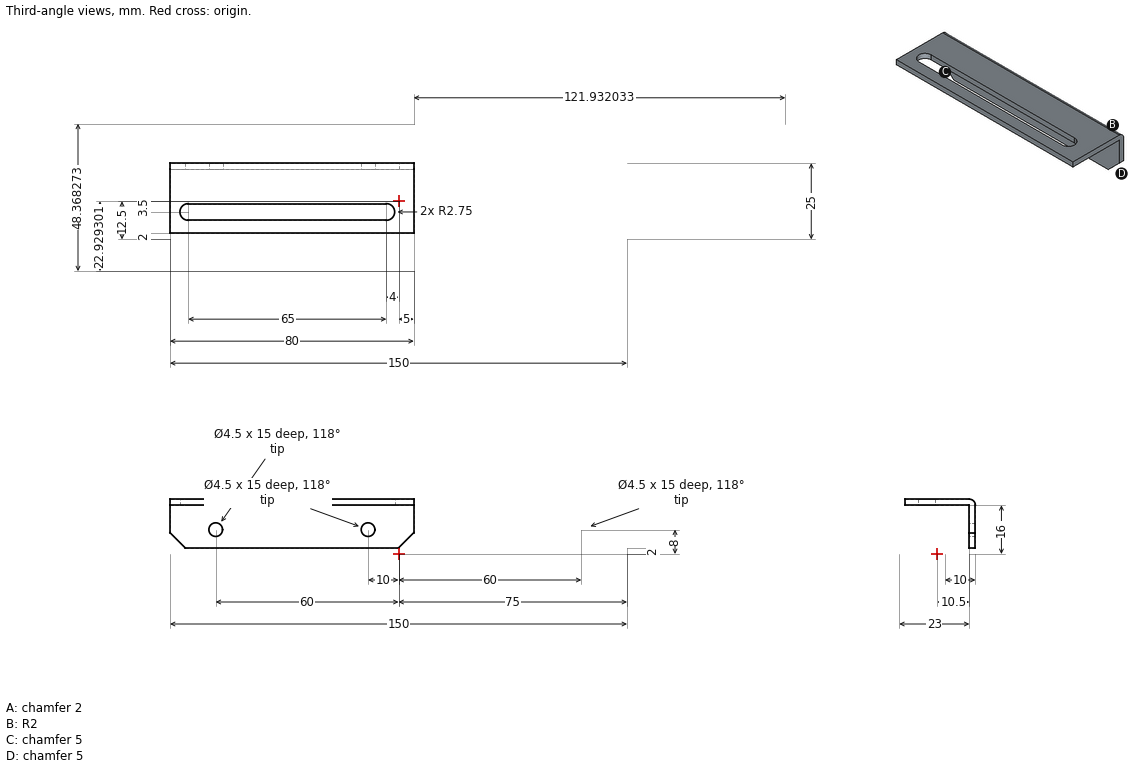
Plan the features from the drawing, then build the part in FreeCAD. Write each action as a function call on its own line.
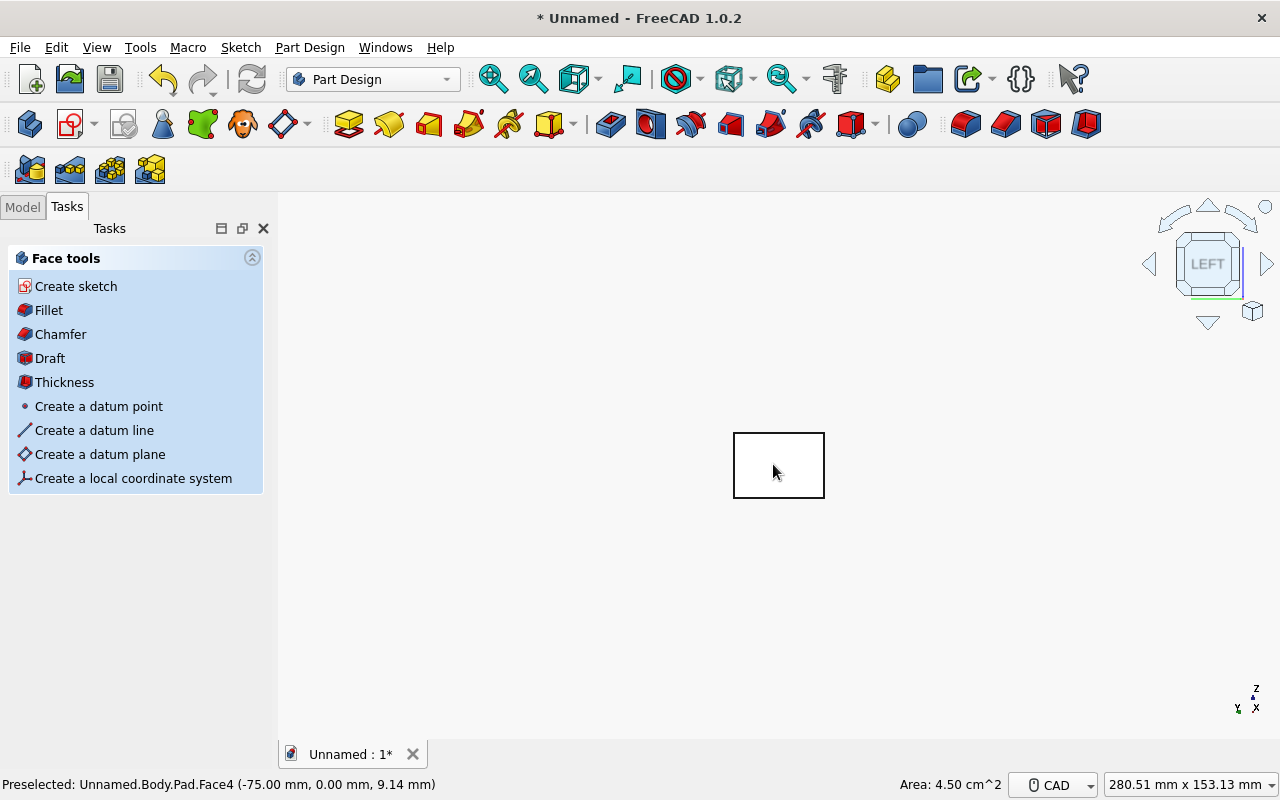
click(70, 124)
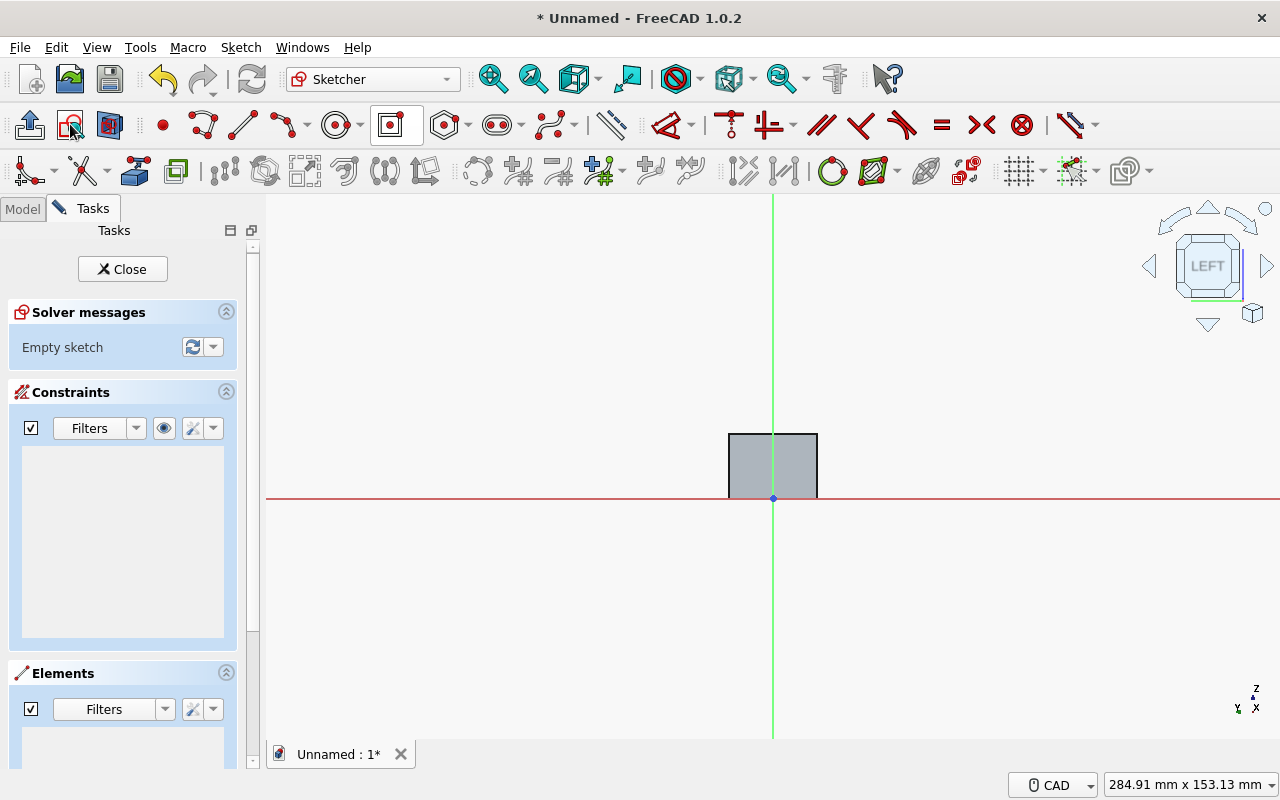
scroll(791, 471, up, 9)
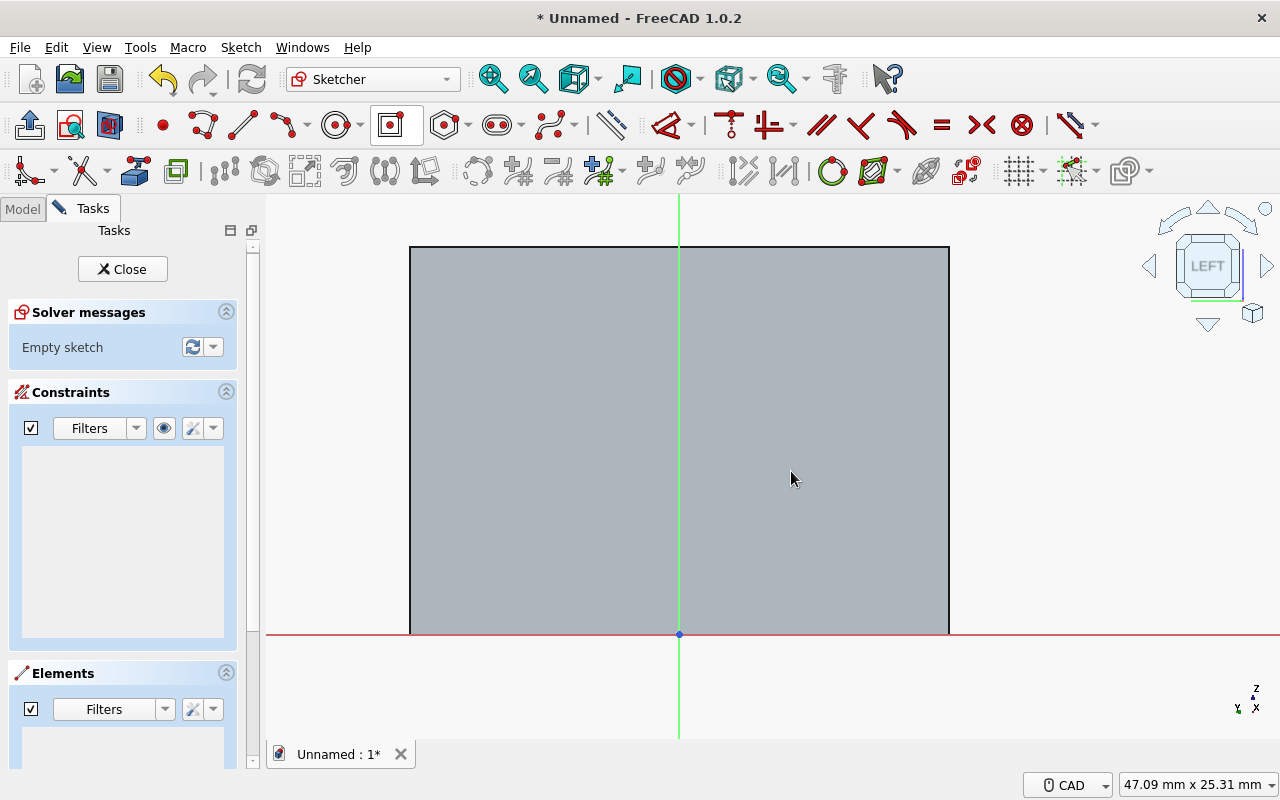
key(g)
key(r)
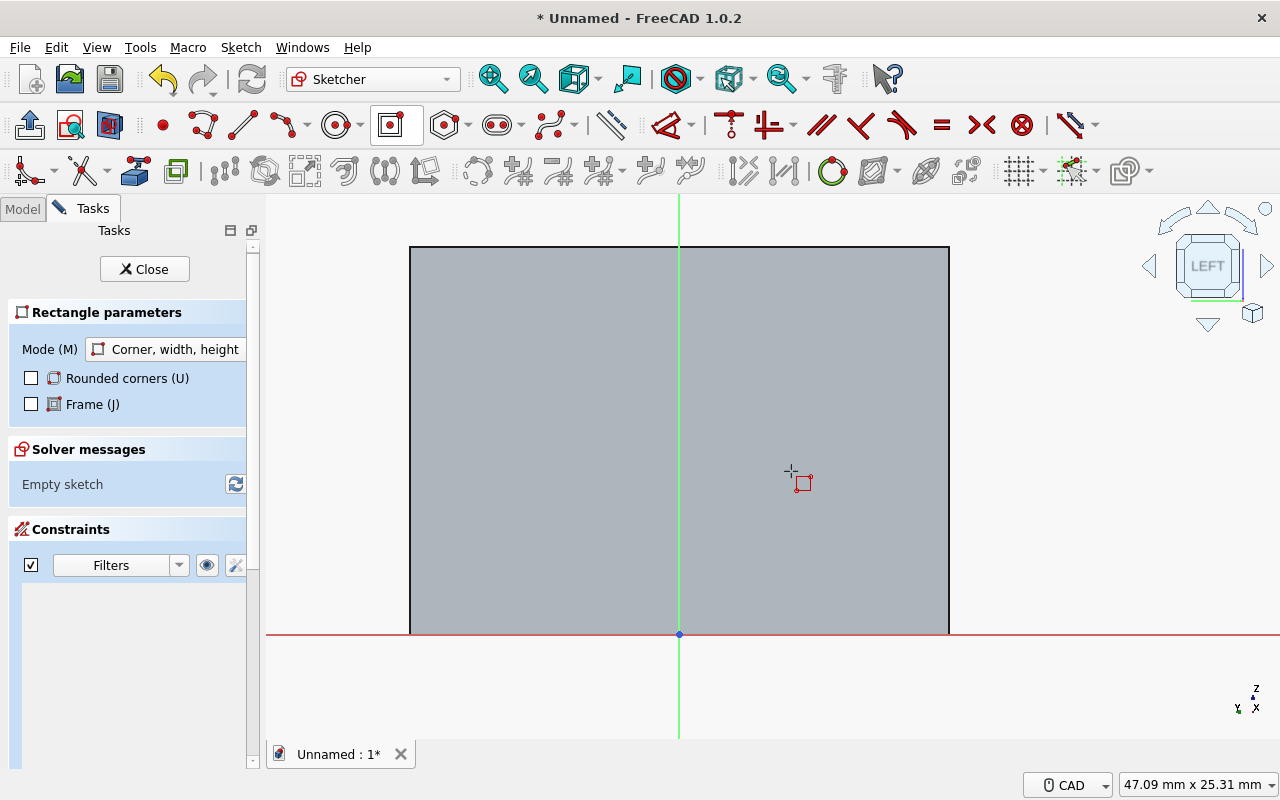
click(453, 290)
click(949, 635)
key(Escape)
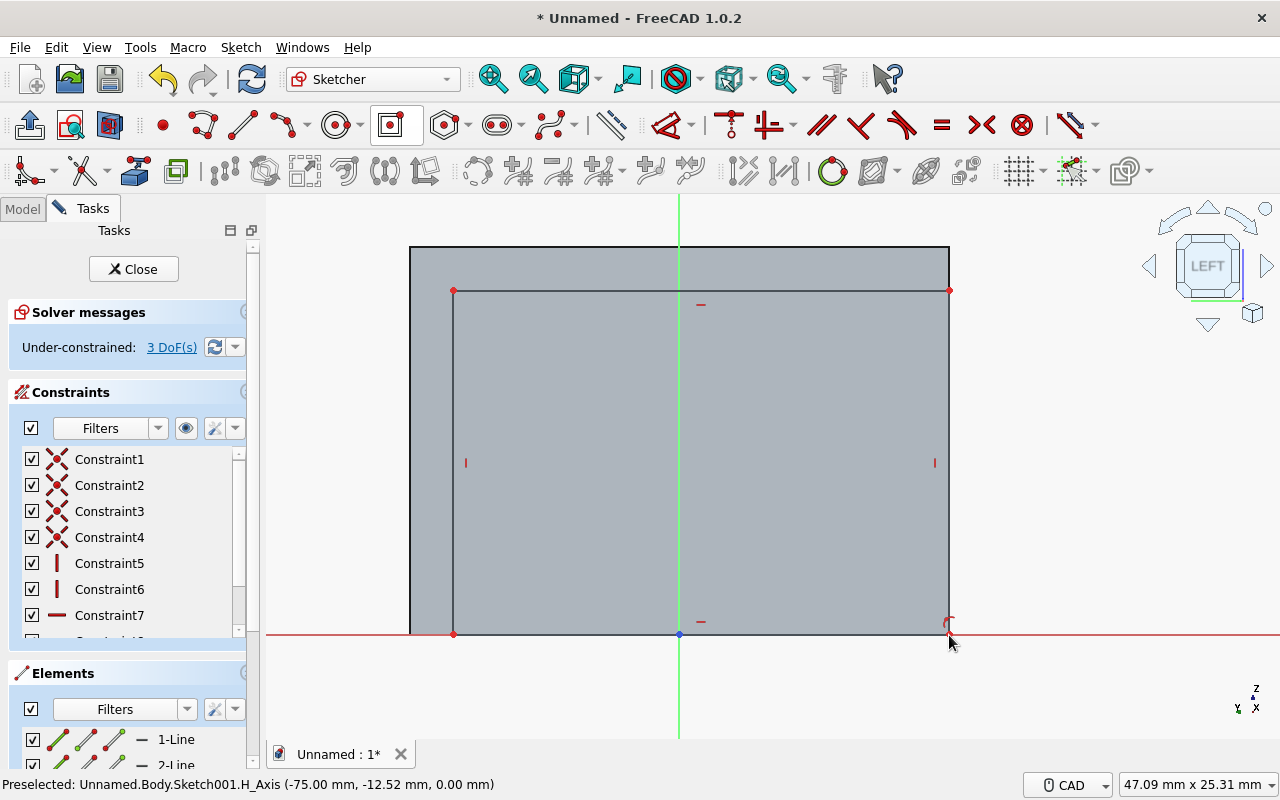
click(666, 126)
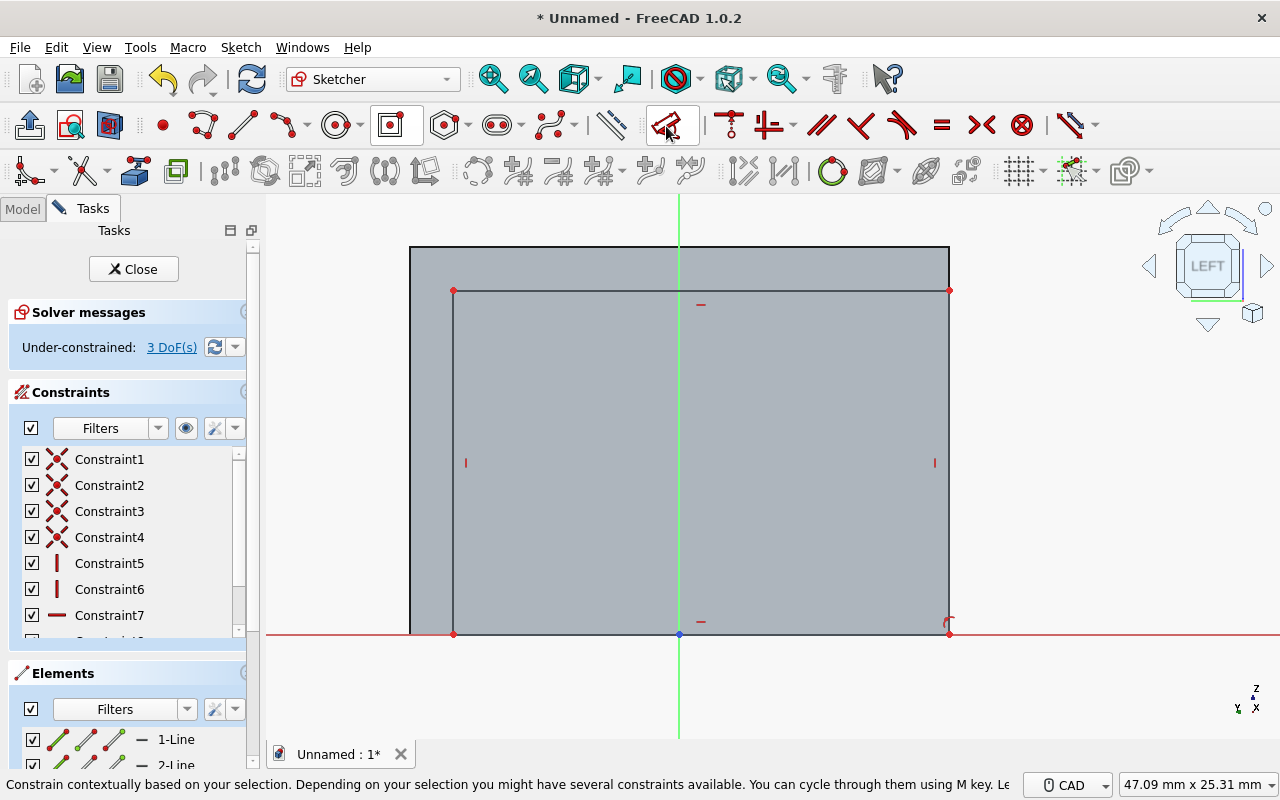
click(453, 394)
click(419, 463)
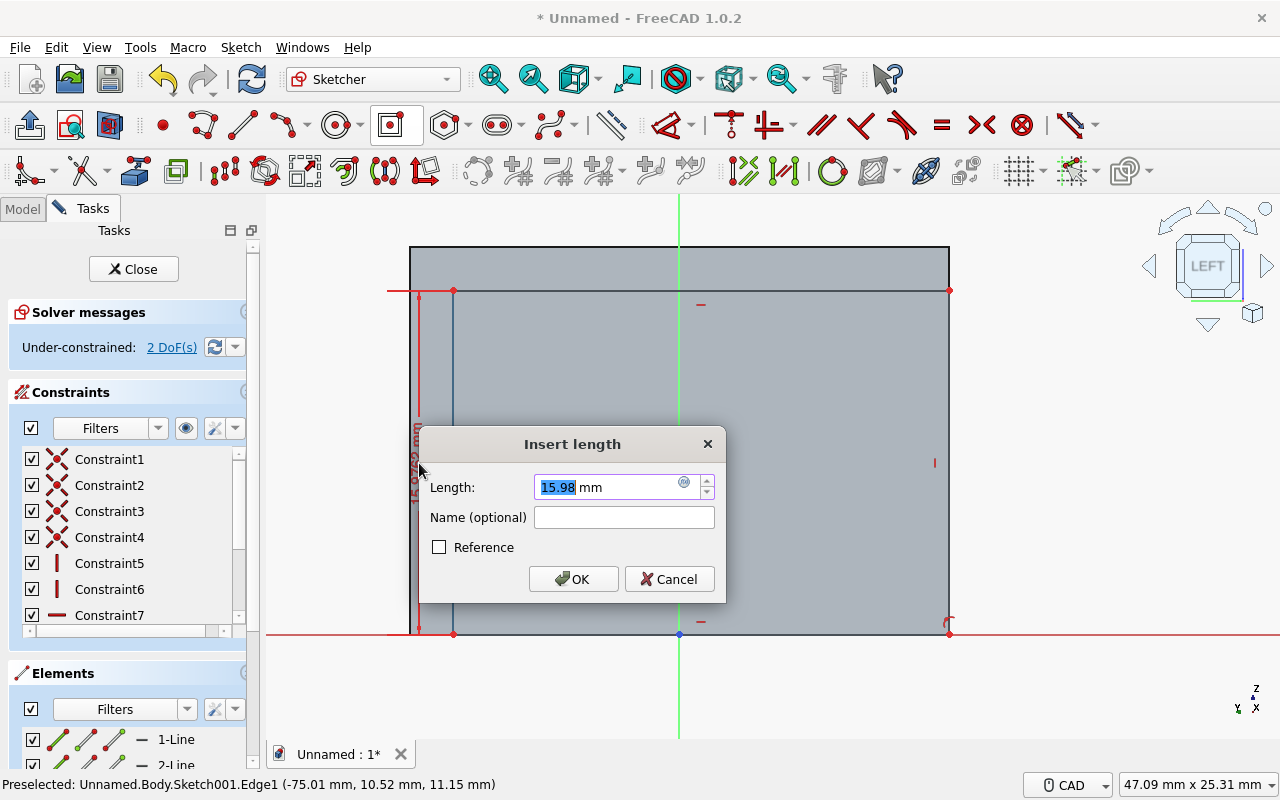
text(16)
key(Return)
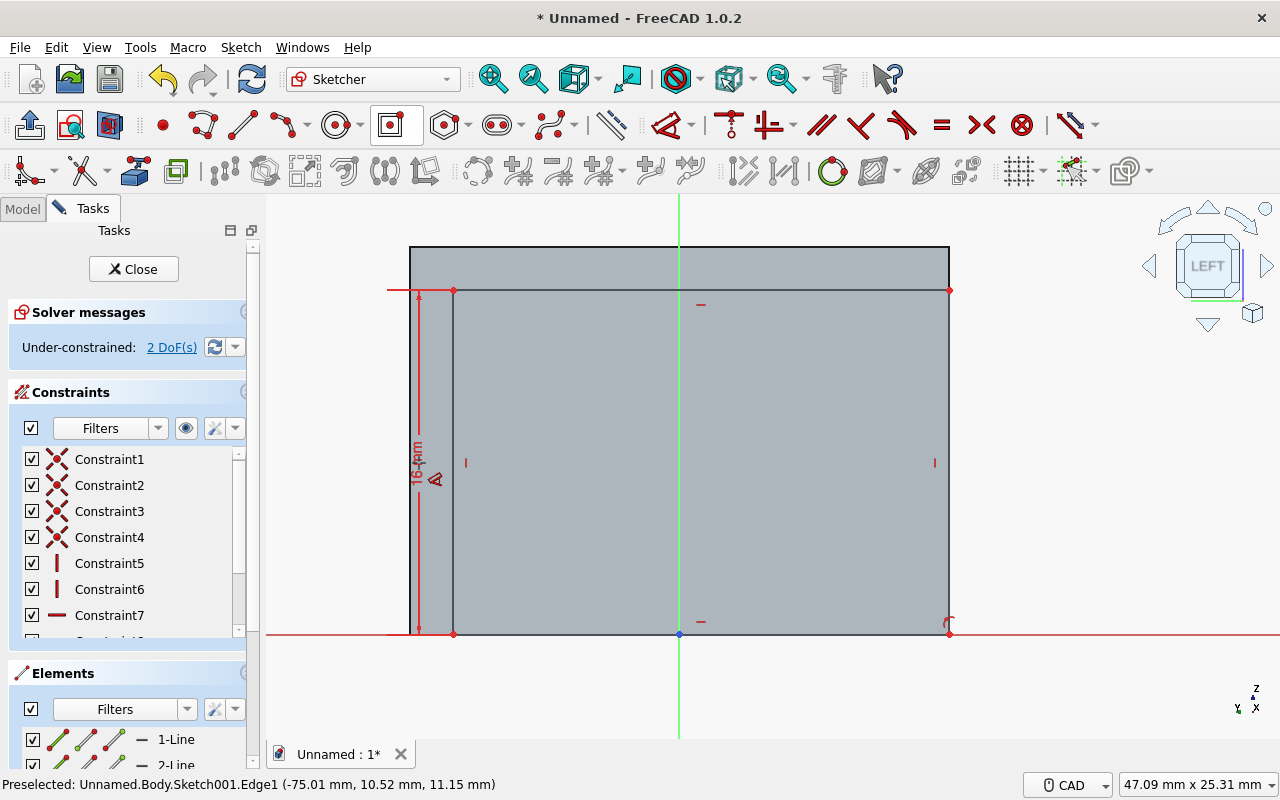
click(602, 635)
click(701, 669)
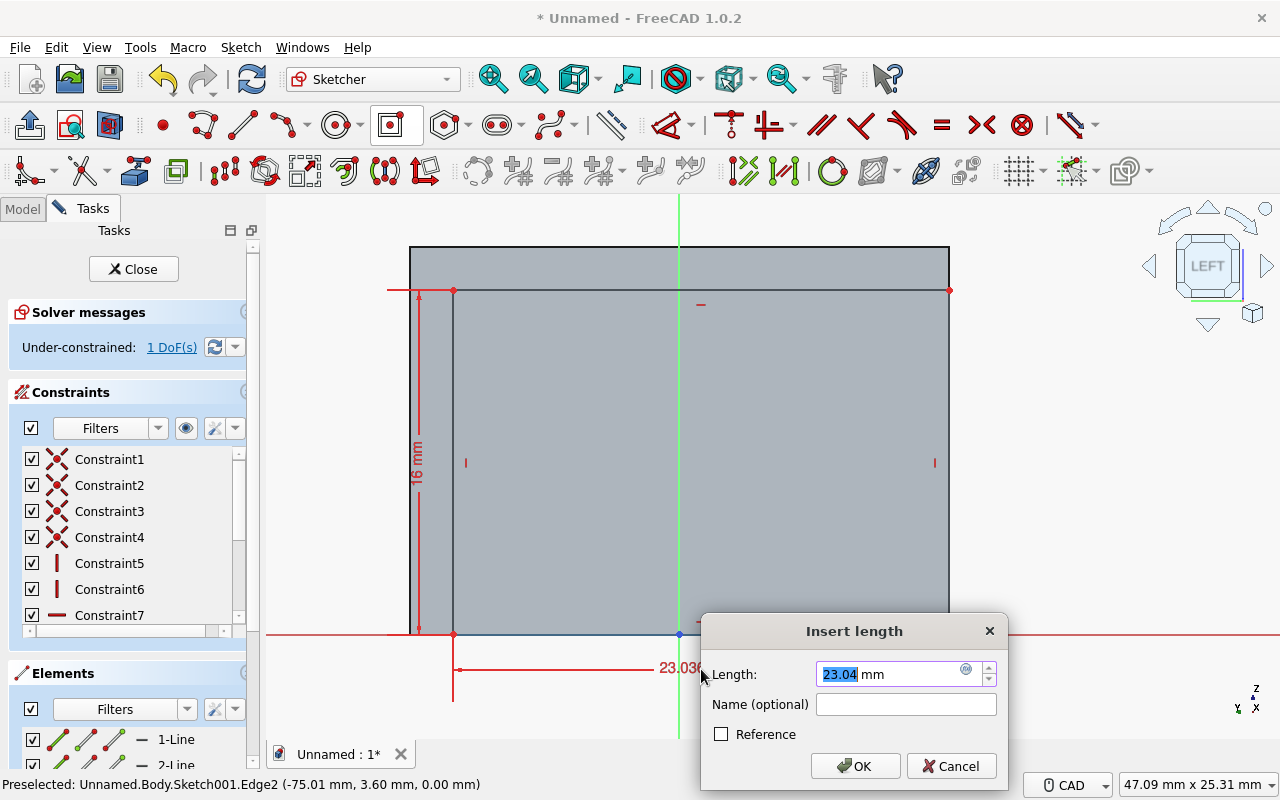
text(23)
key(Return)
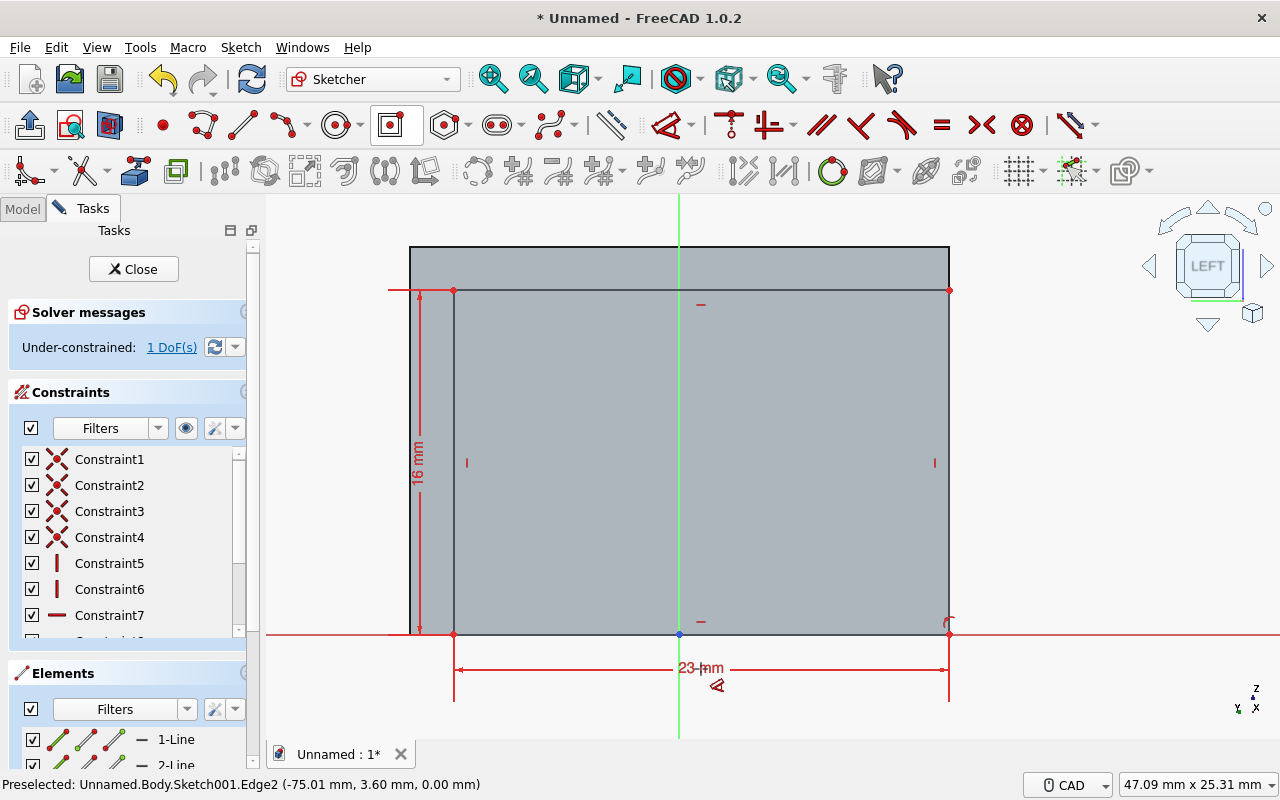
click(454, 290)
click(567, 669)